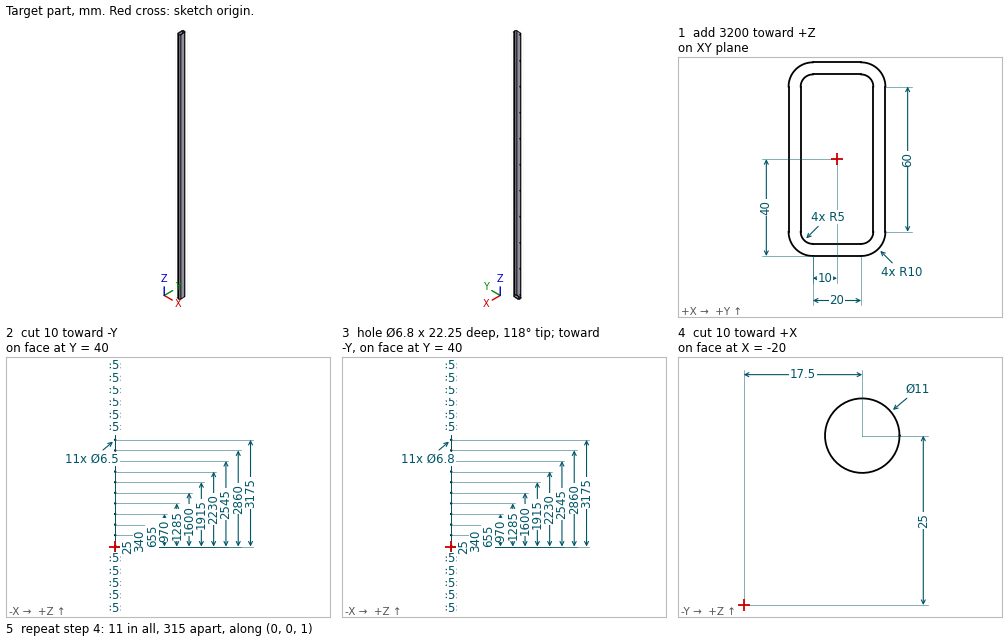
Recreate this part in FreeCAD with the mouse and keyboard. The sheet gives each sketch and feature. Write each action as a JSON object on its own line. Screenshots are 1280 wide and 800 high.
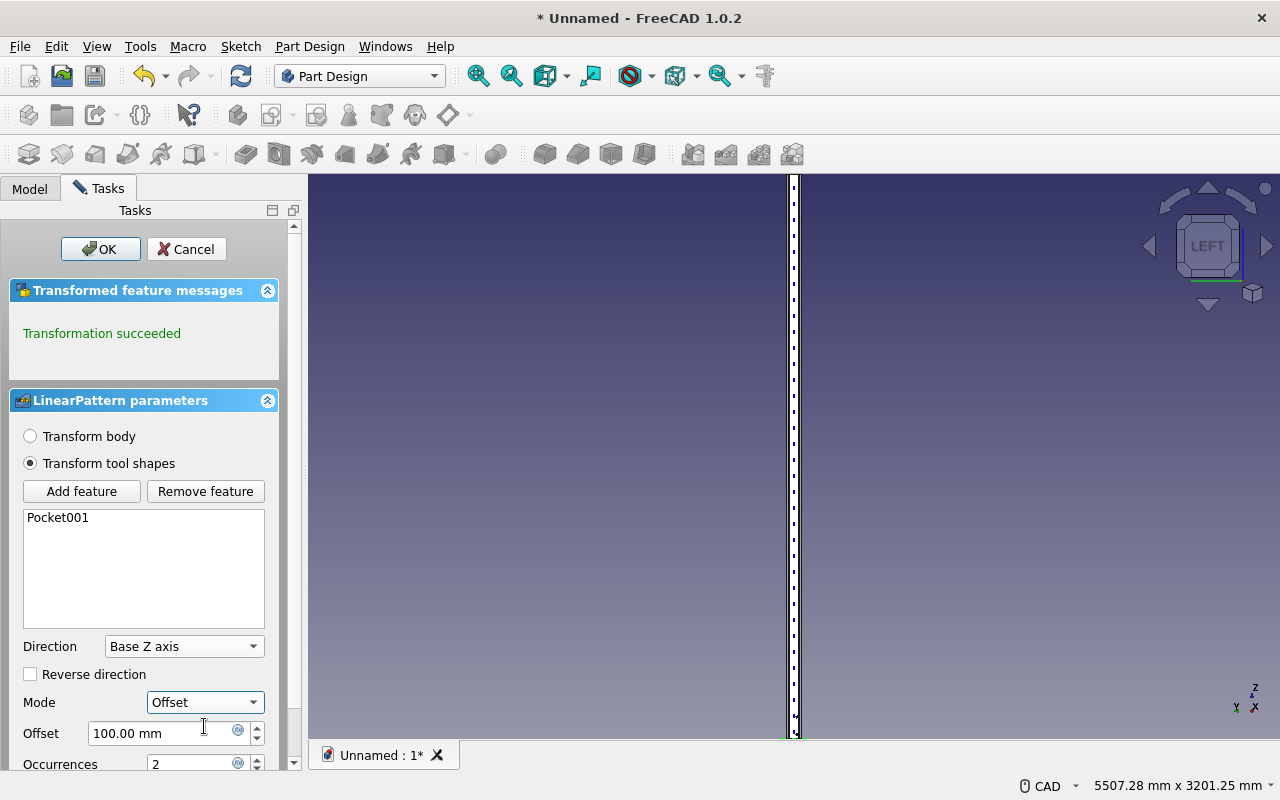
{"action": "triple_click", "coordinate": [170, 734]}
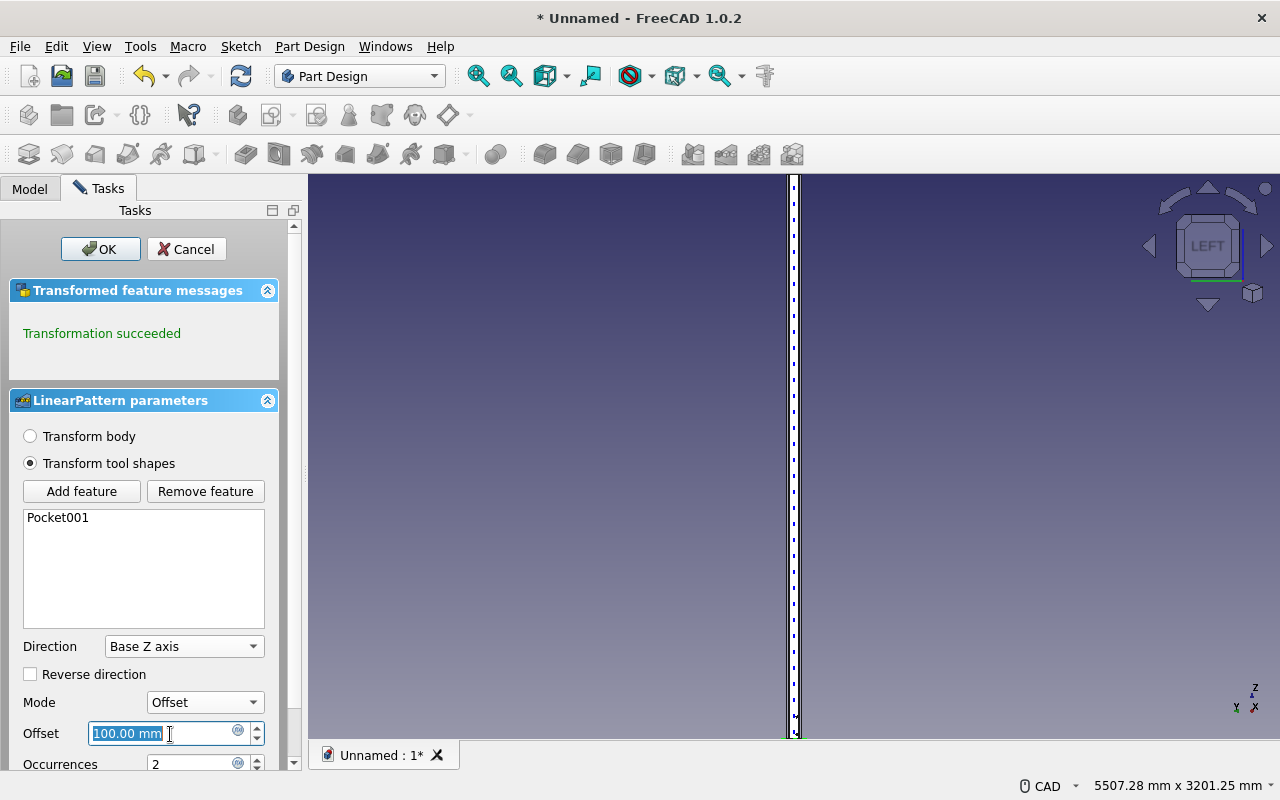
{"action": "type", "text": "315"}
{"action": "key", "text": "Tab"}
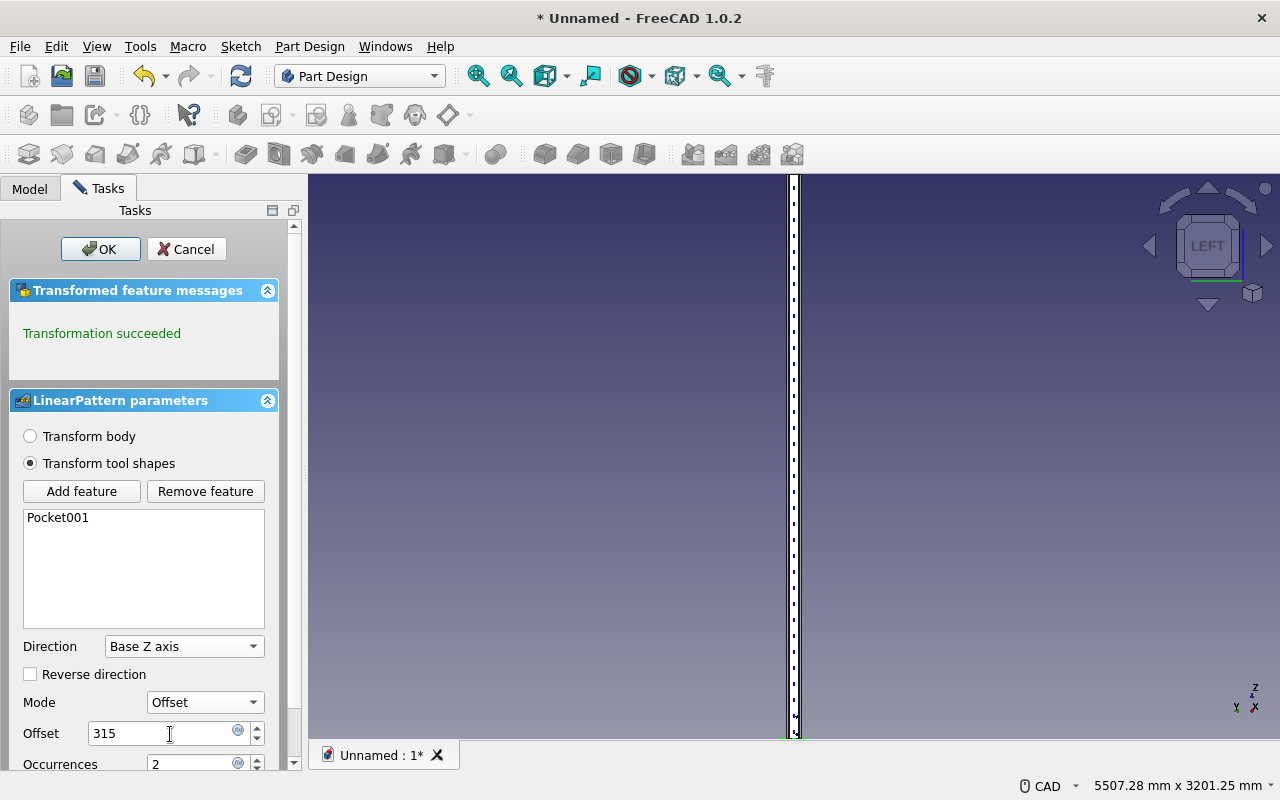
{"action": "scroll", "coordinate": [294, 495], "scroll_direction": "down", "scroll_amount": 2}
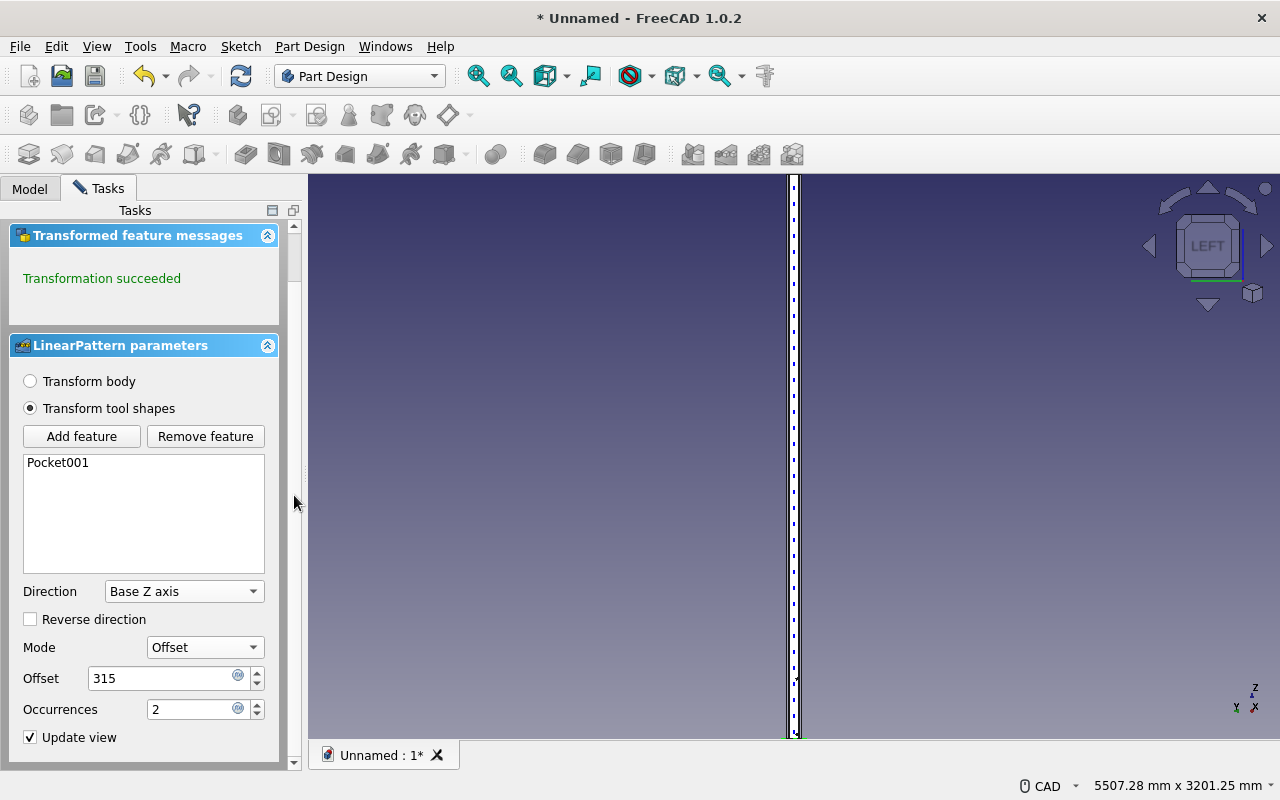
{"action": "triple_click", "coordinate": [199, 710]}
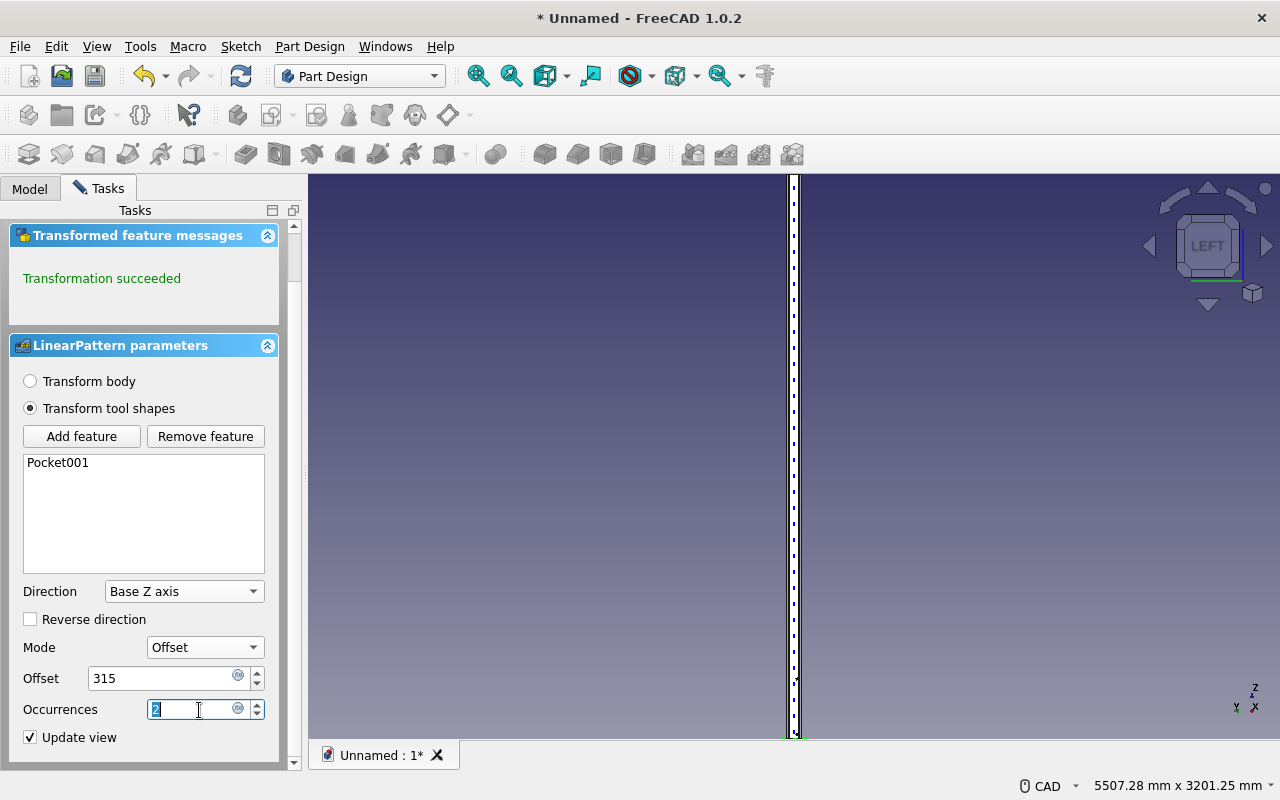
{"action": "type", "text": "11"}
{"action": "key", "text": "Tab"}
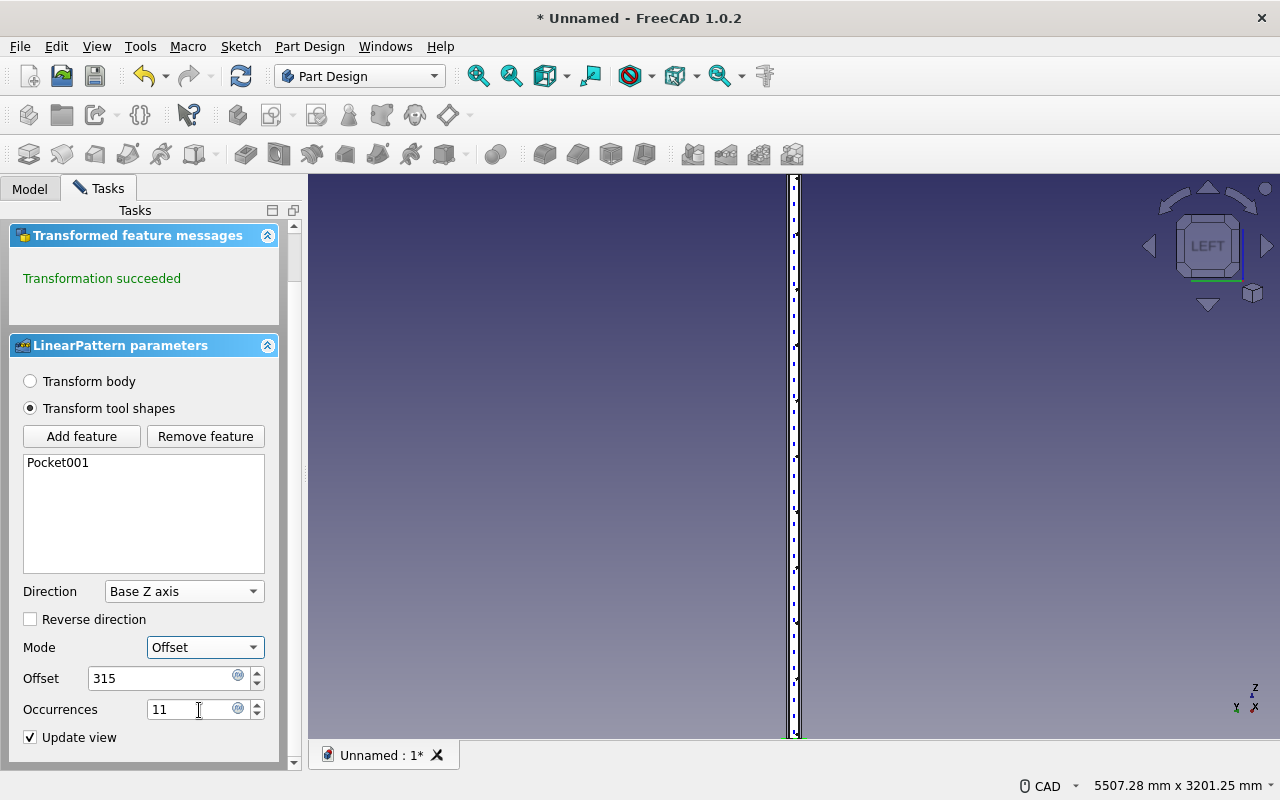
{"action": "scroll", "coordinate": [294, 495], "scroll_direction": "up", "scroll_amount": 2}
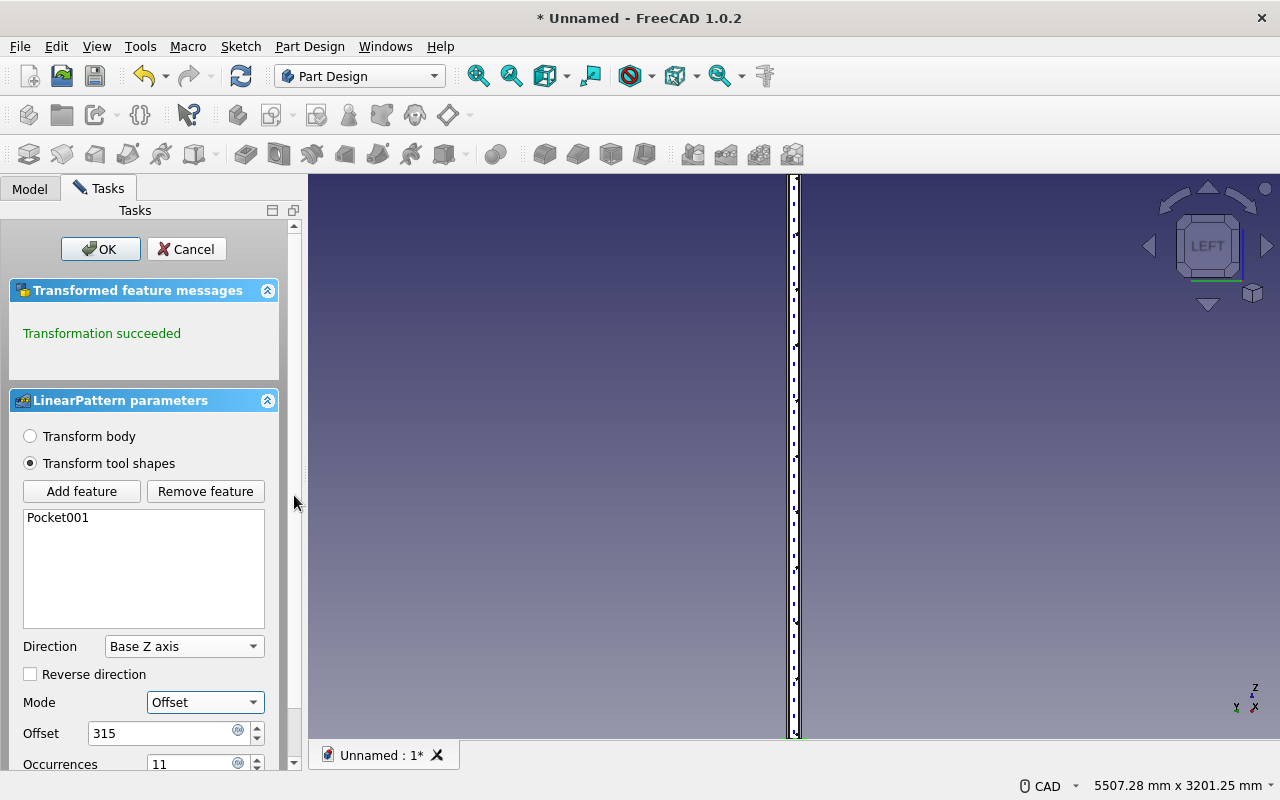
{"action": "left_click", "coordinate": [101, 249]}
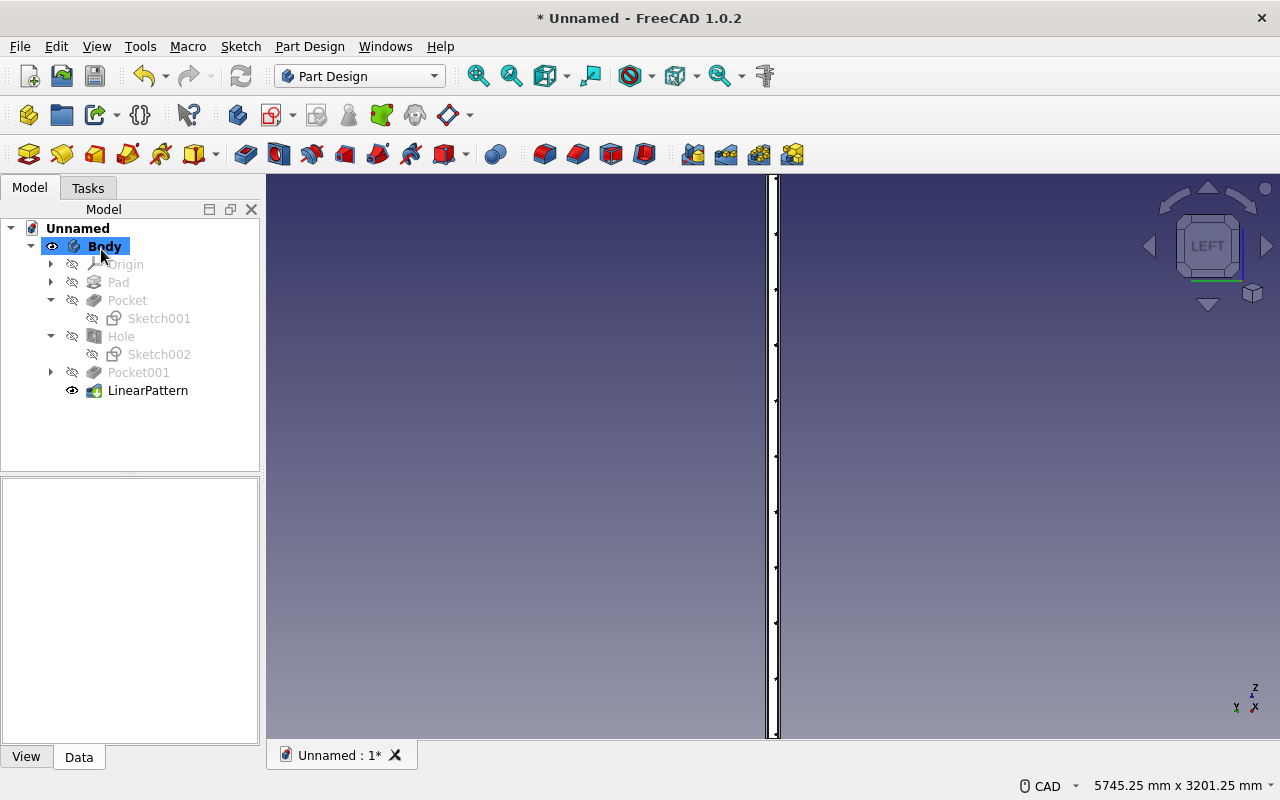
{"action": "key", "text": "0"}